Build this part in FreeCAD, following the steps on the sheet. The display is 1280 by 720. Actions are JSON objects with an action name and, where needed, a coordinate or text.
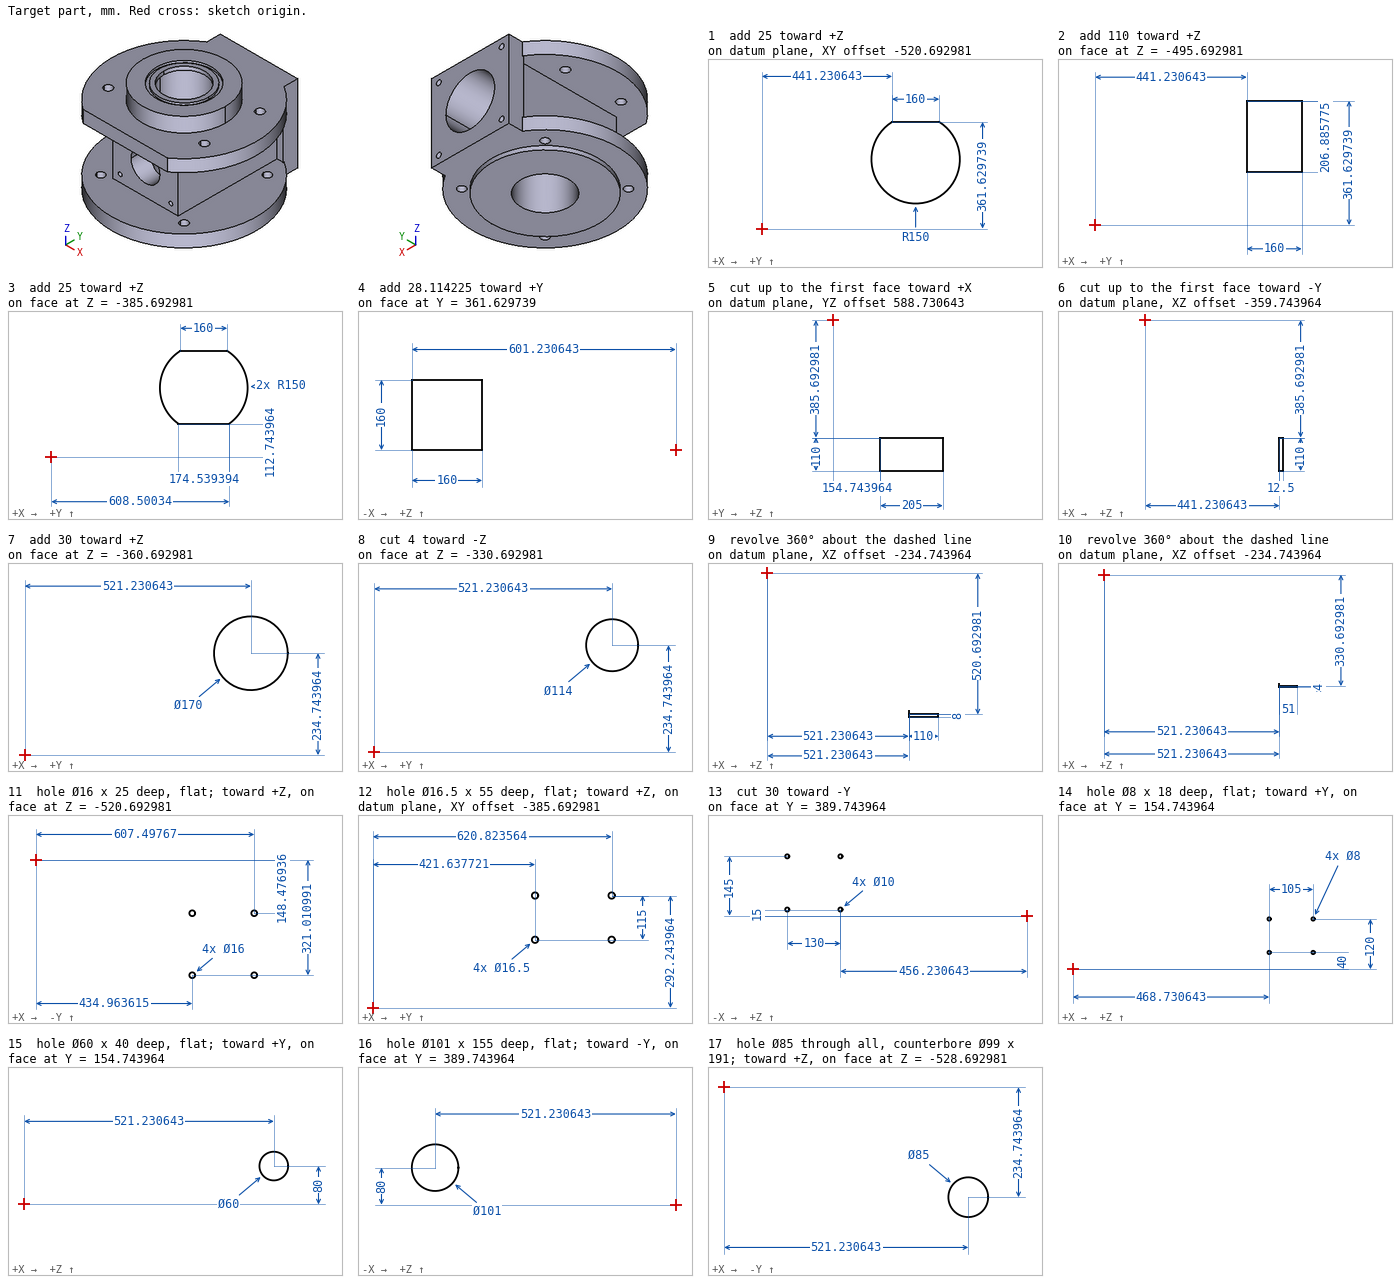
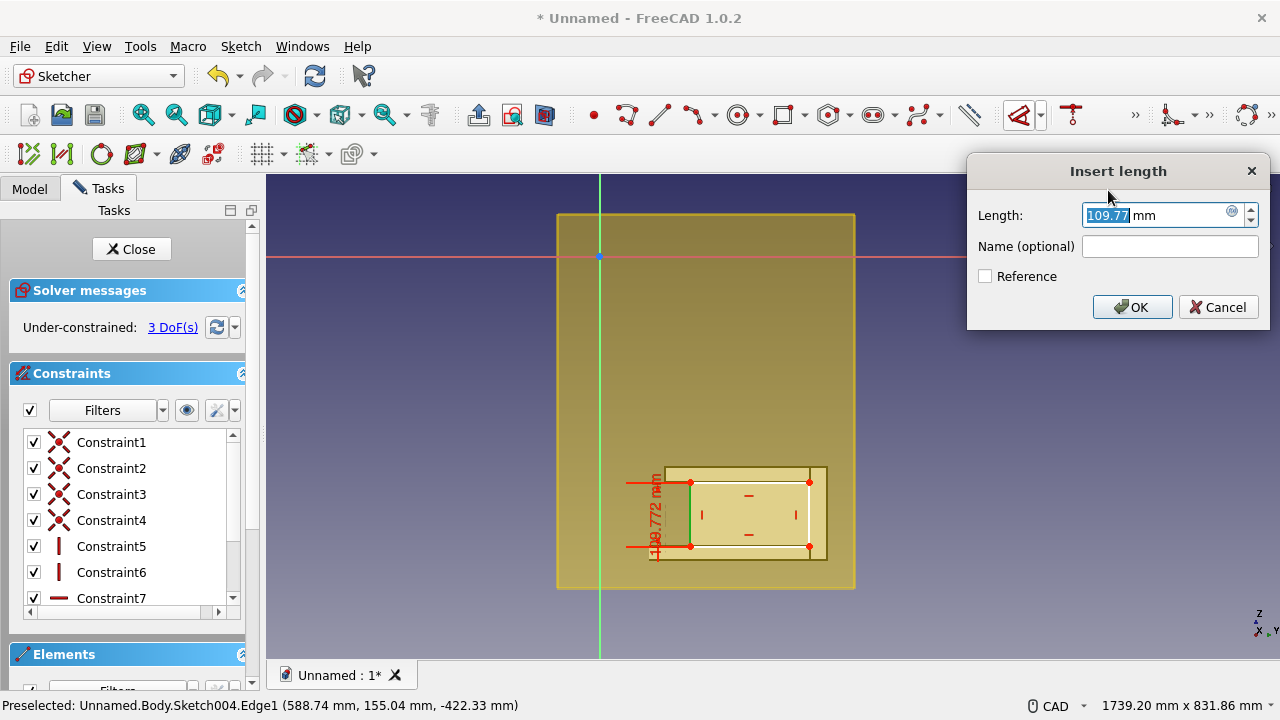
{"action": "type", "text": "110"}
{"action": "key", "text": "Return"}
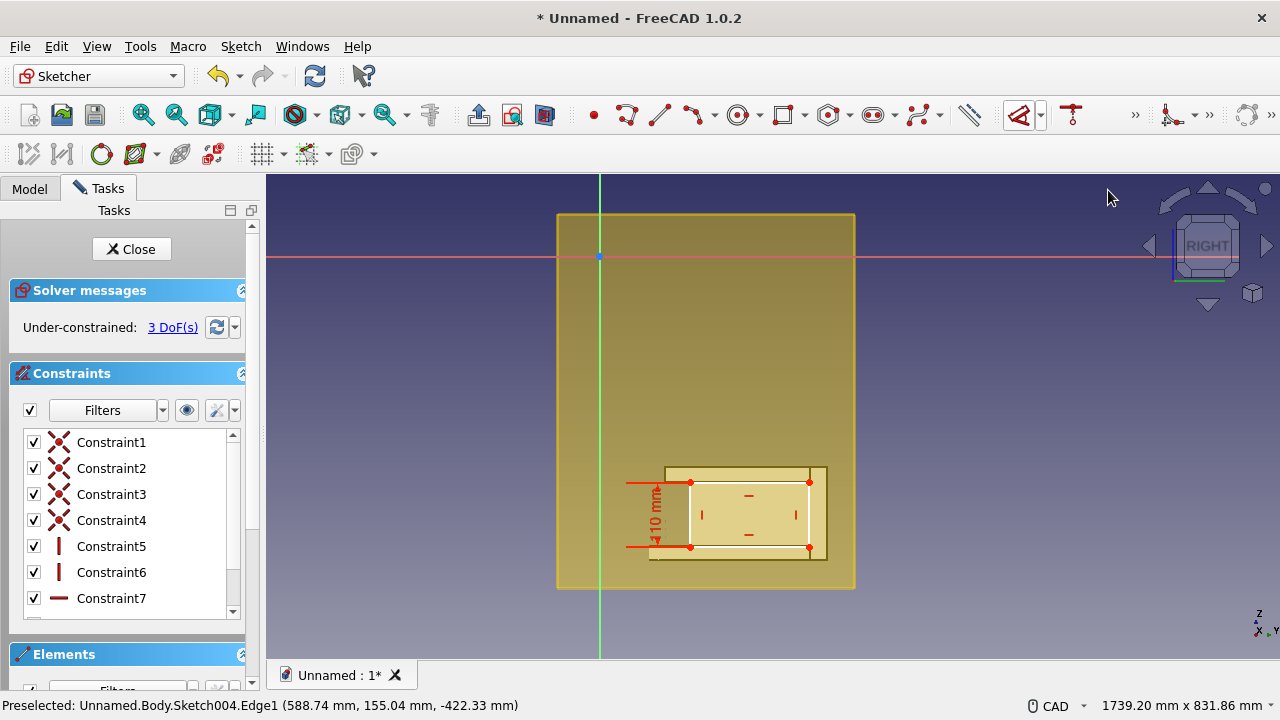
{"action": "left_click", "coordinate": [726, 547]}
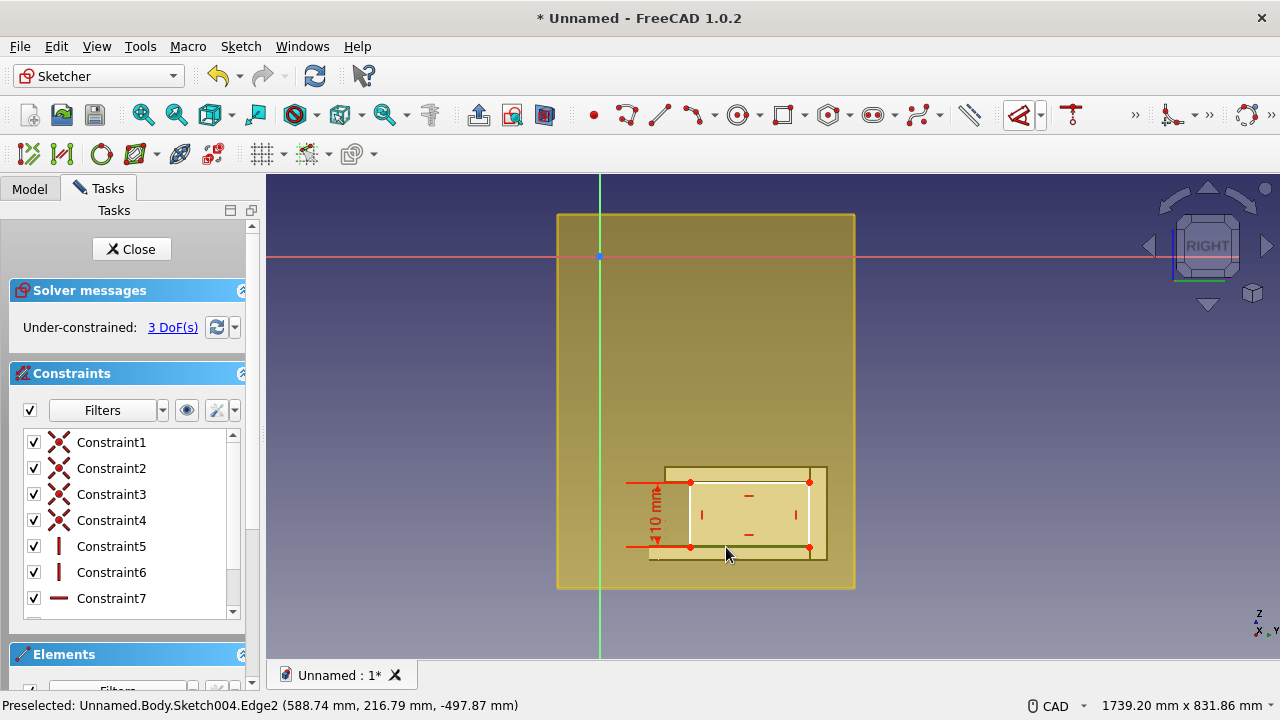
{"action": "key", "text": "l"}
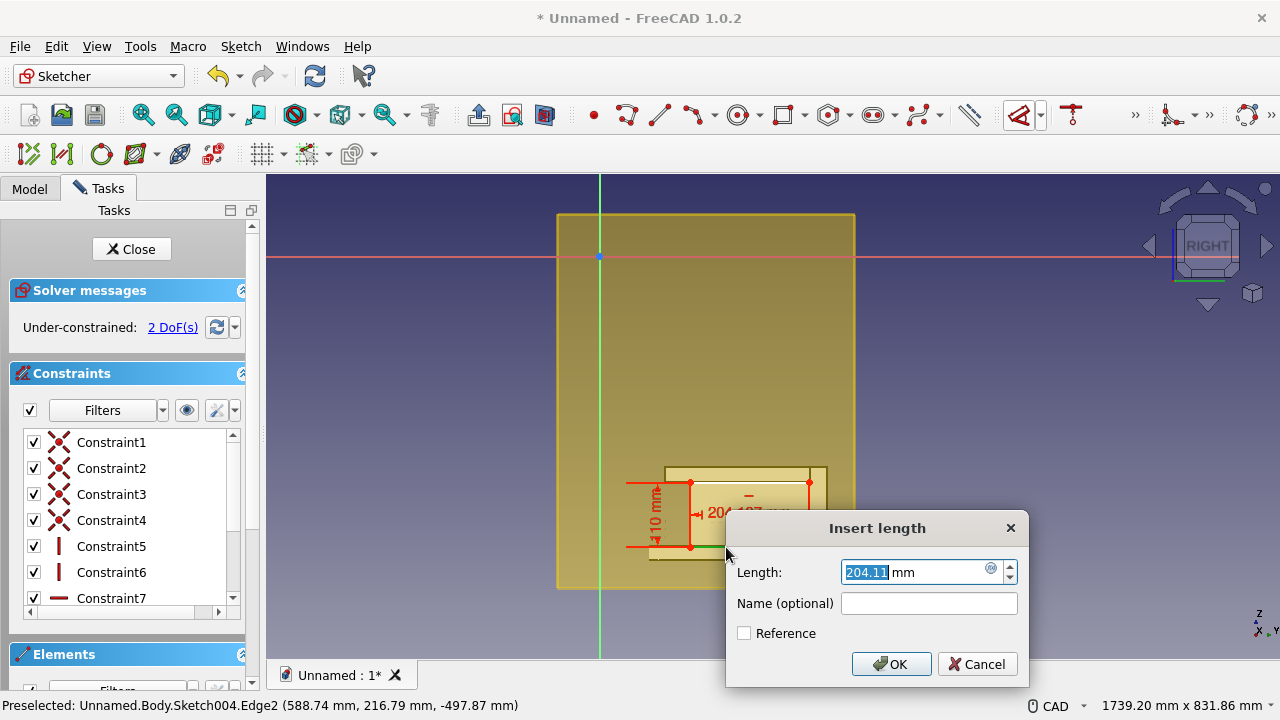
{"action": "type", "text": "205"}
{"action": "key", "text": "Return"}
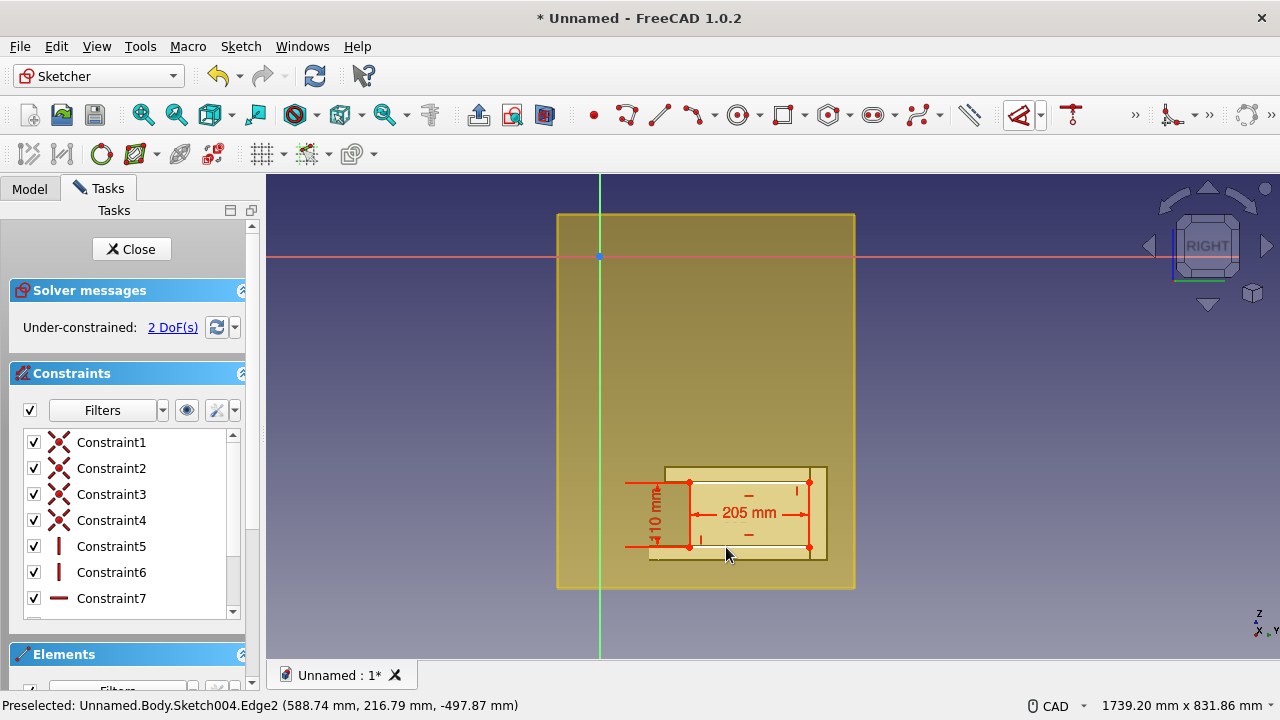
{"action": "left_click", "coordinate": [690, 483]}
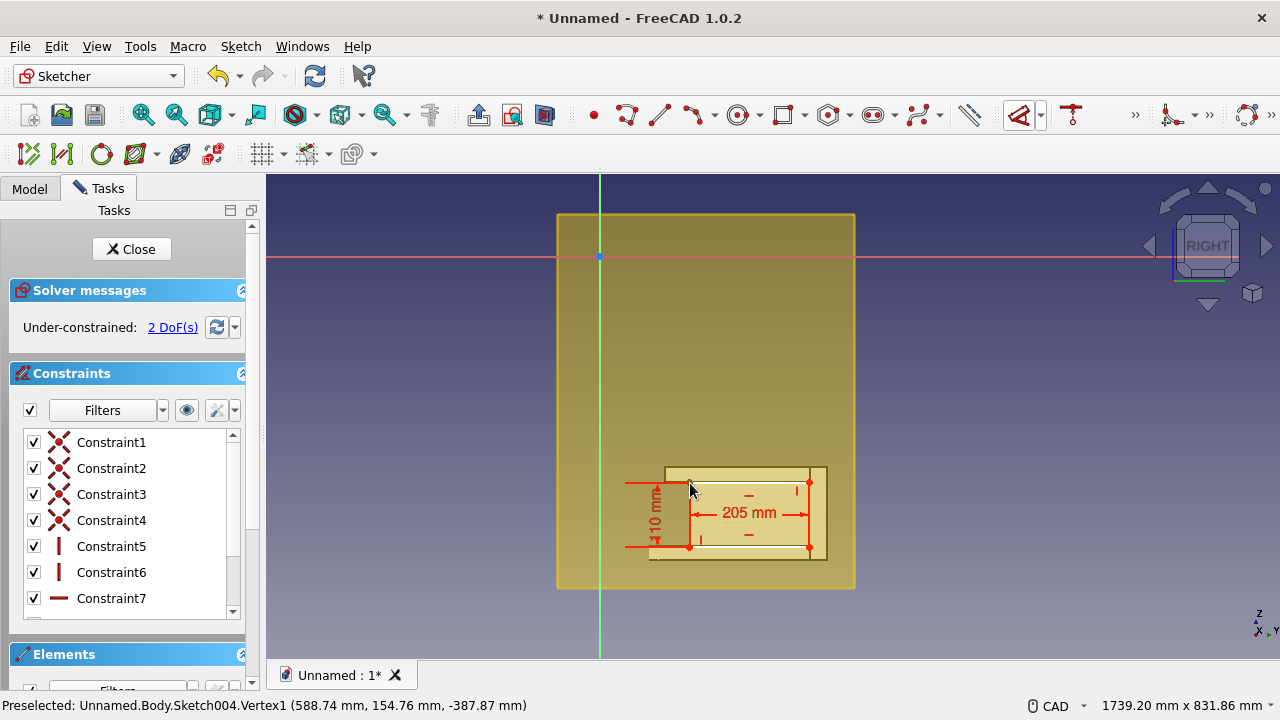
{"action": "left_click", "coordinate": [1040, 116]}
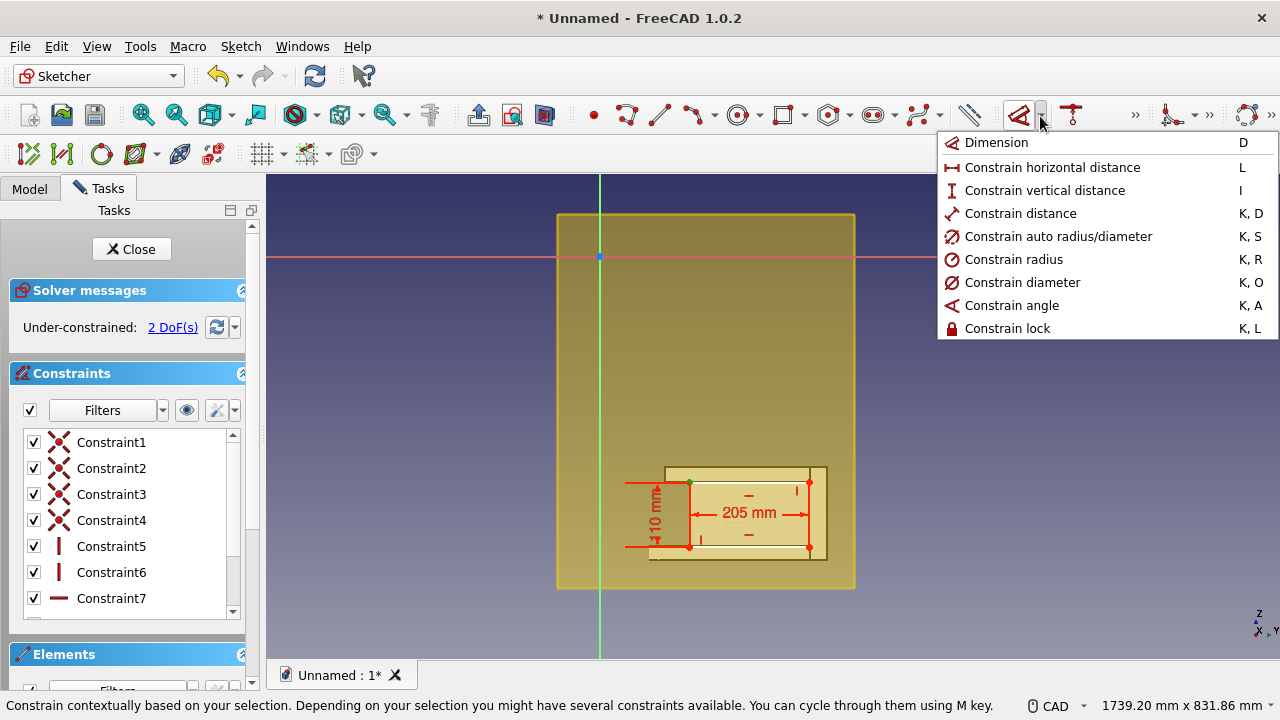
{"action": "left_click", "coordinate": [1108, 168]}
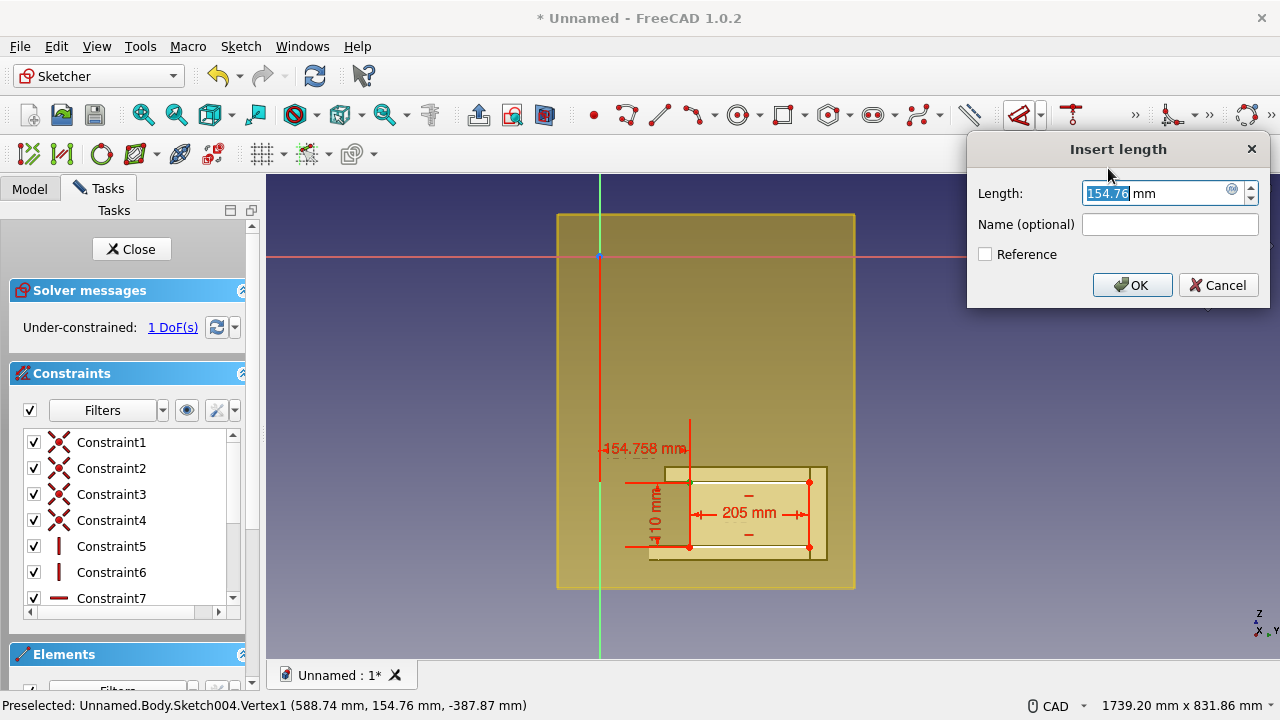
{"action": "type", "text": "154.743964"}
{"action": "key", "text": "Return"}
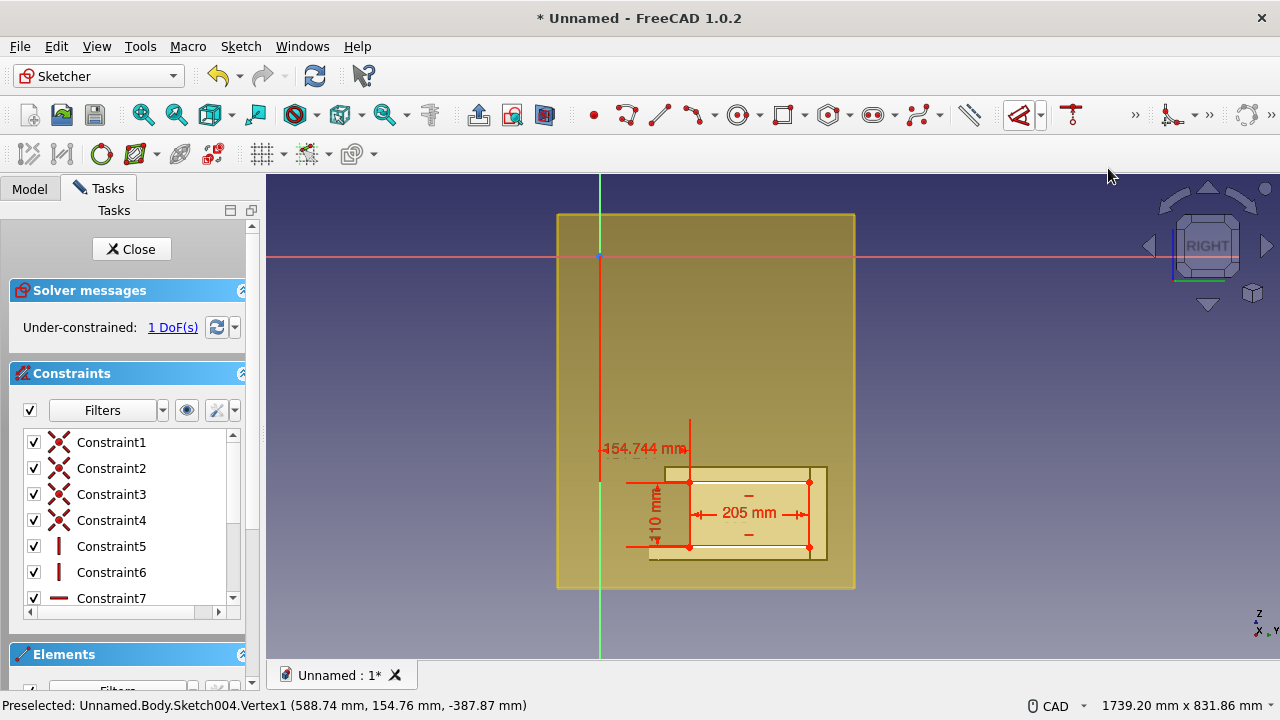
{"action": "left_click", "coordinate": [690, 483]}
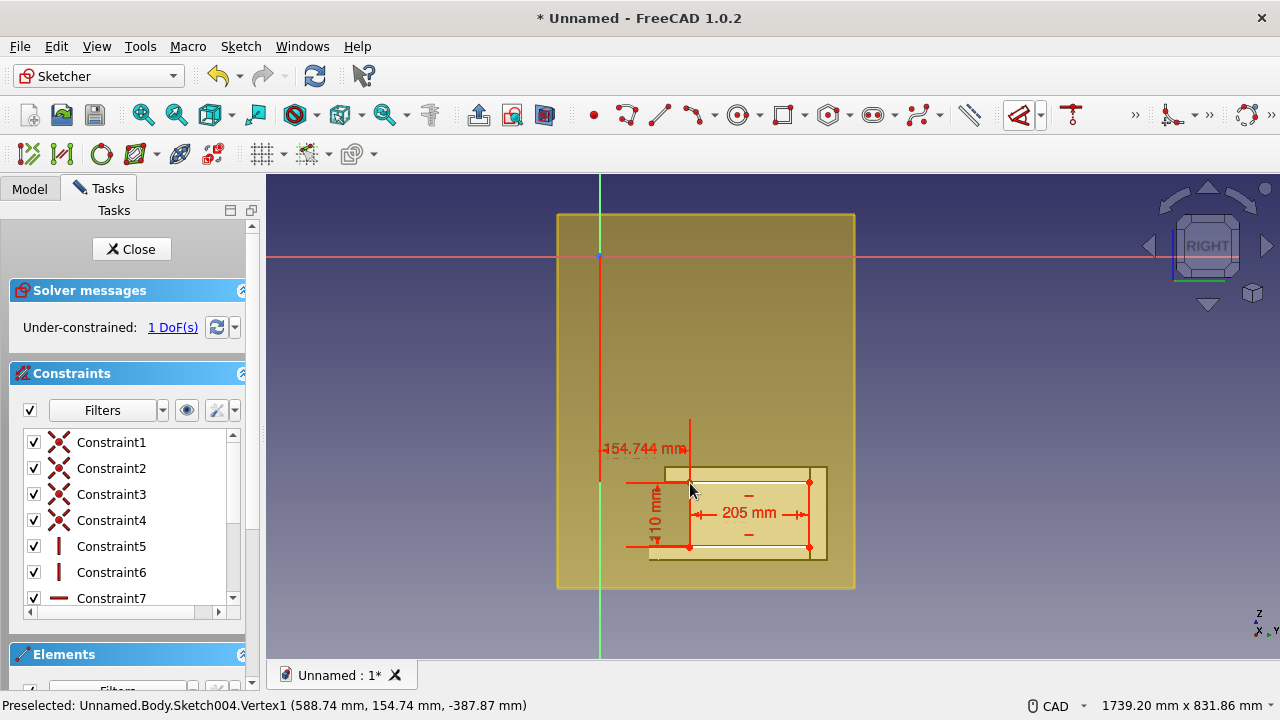
{"action": "left_click", "coordinate": [1040, 116]}